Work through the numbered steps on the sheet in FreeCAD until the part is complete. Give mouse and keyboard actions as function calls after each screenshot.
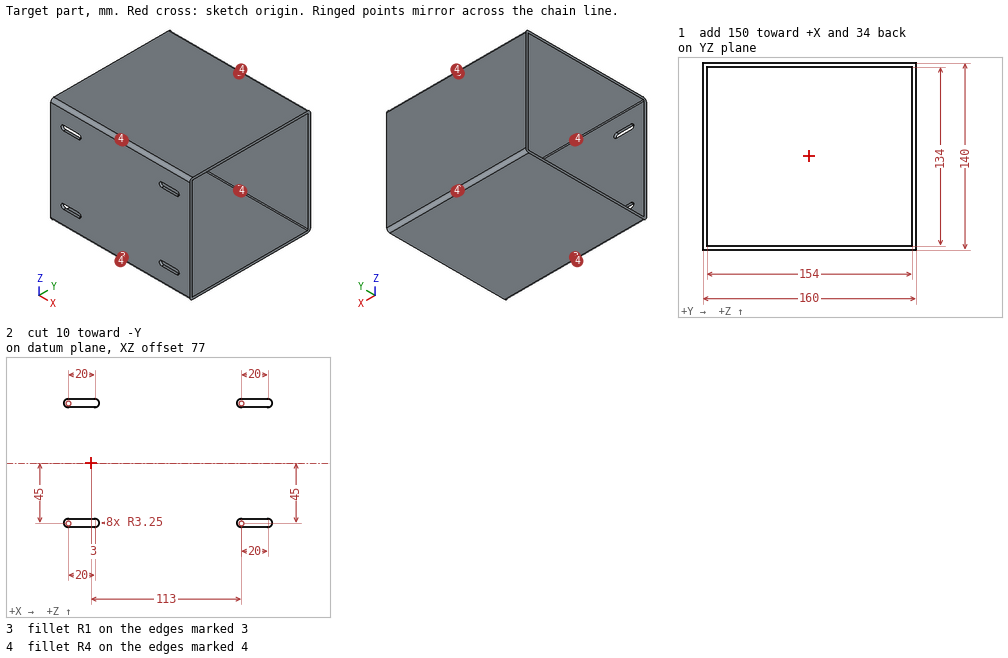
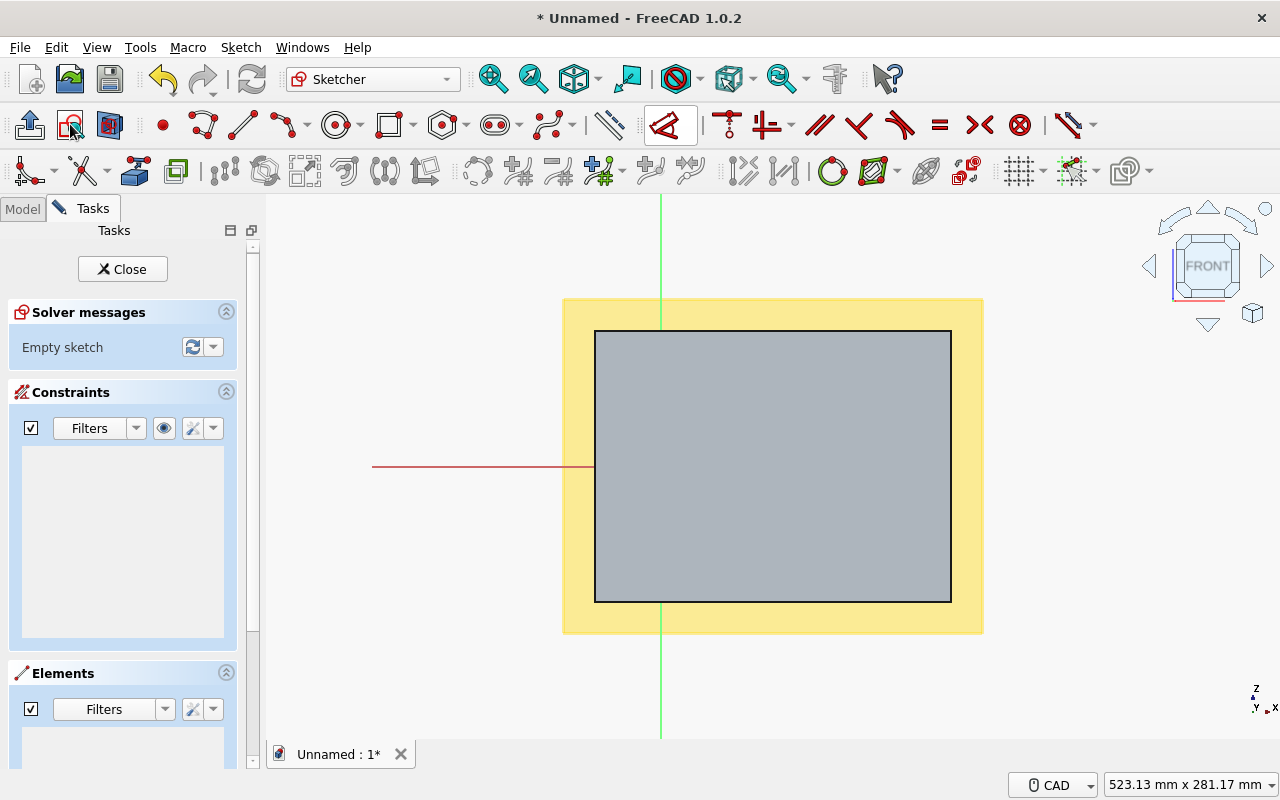
key(q)
key(s)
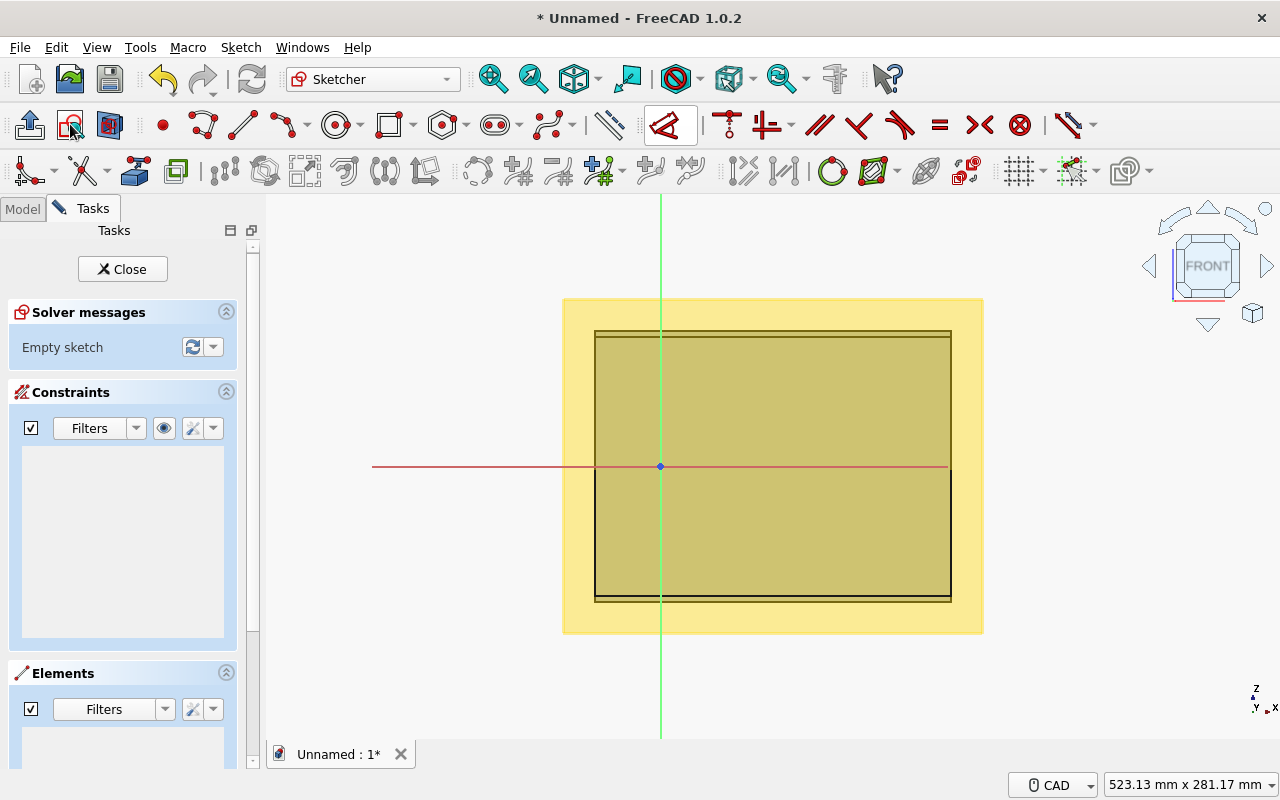
scroll(856, 466, up, 3)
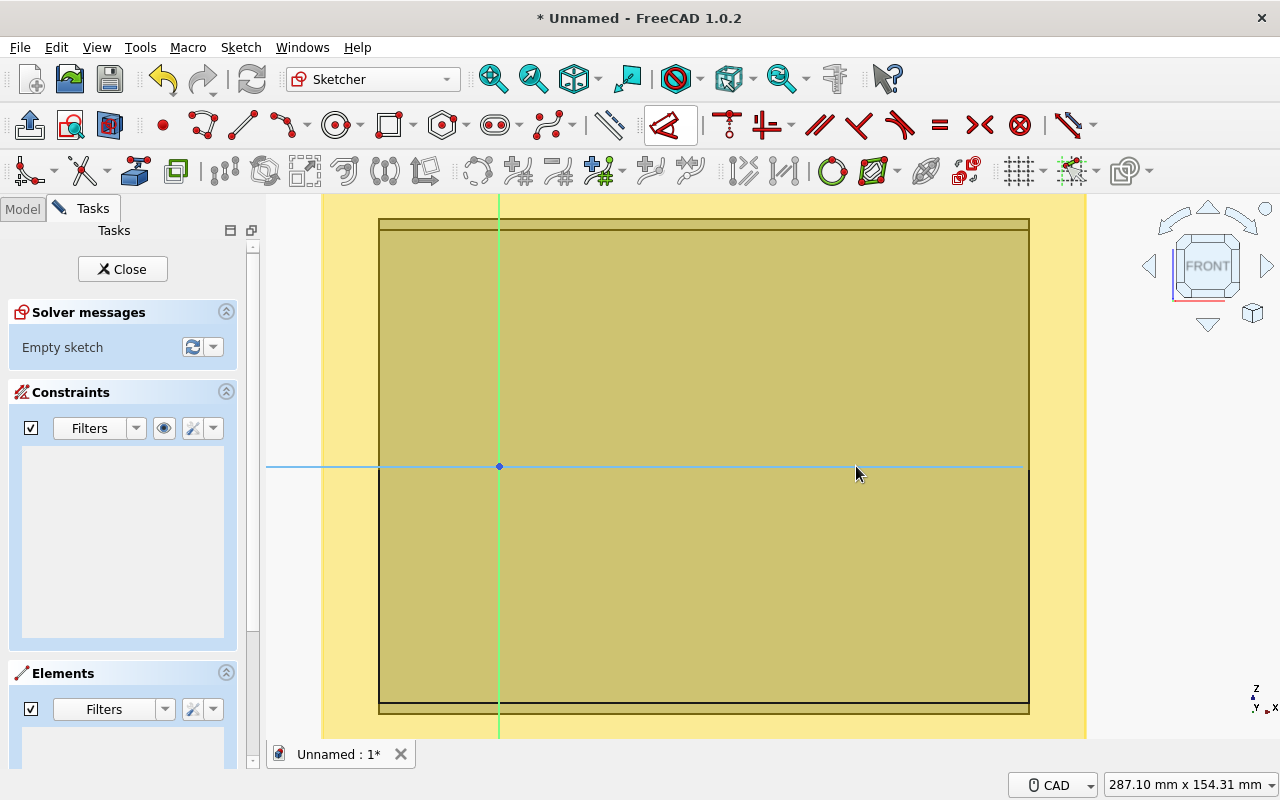
click(496, 126)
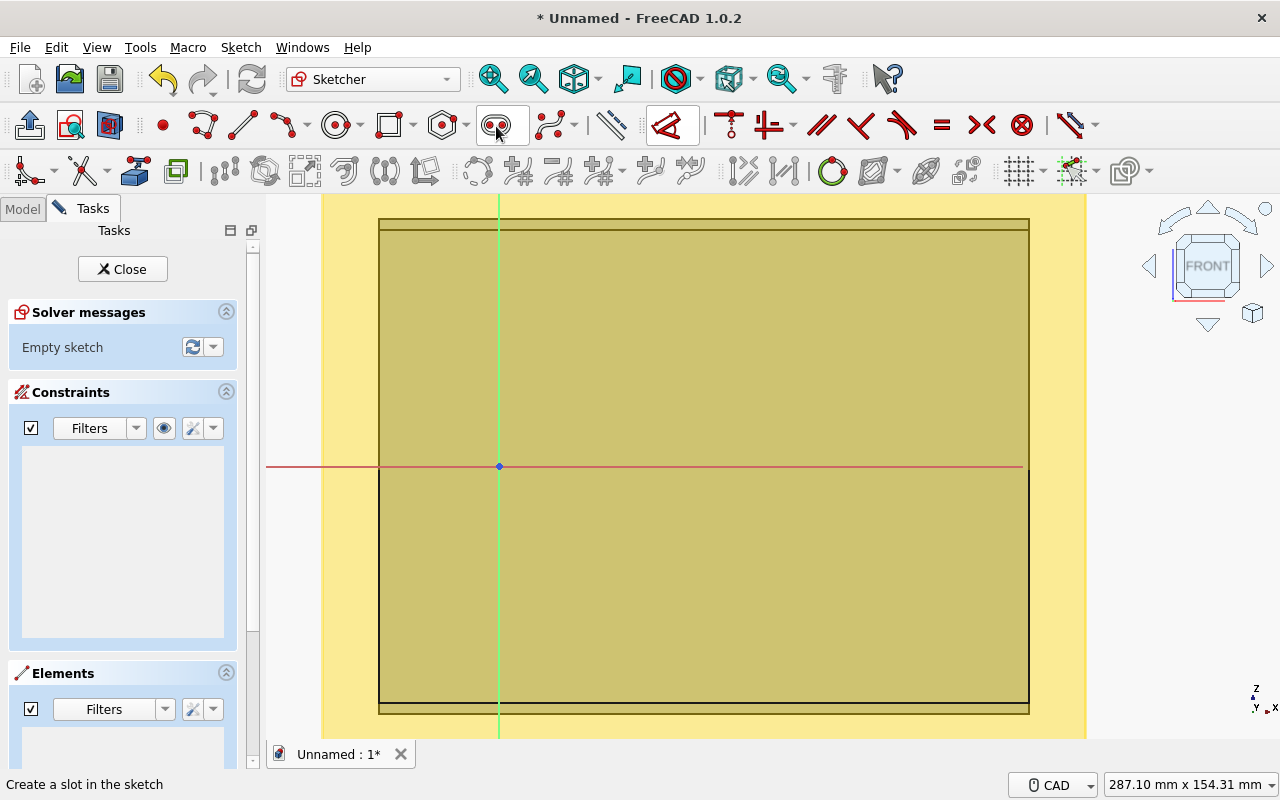
scroll(439, 625, up, 4)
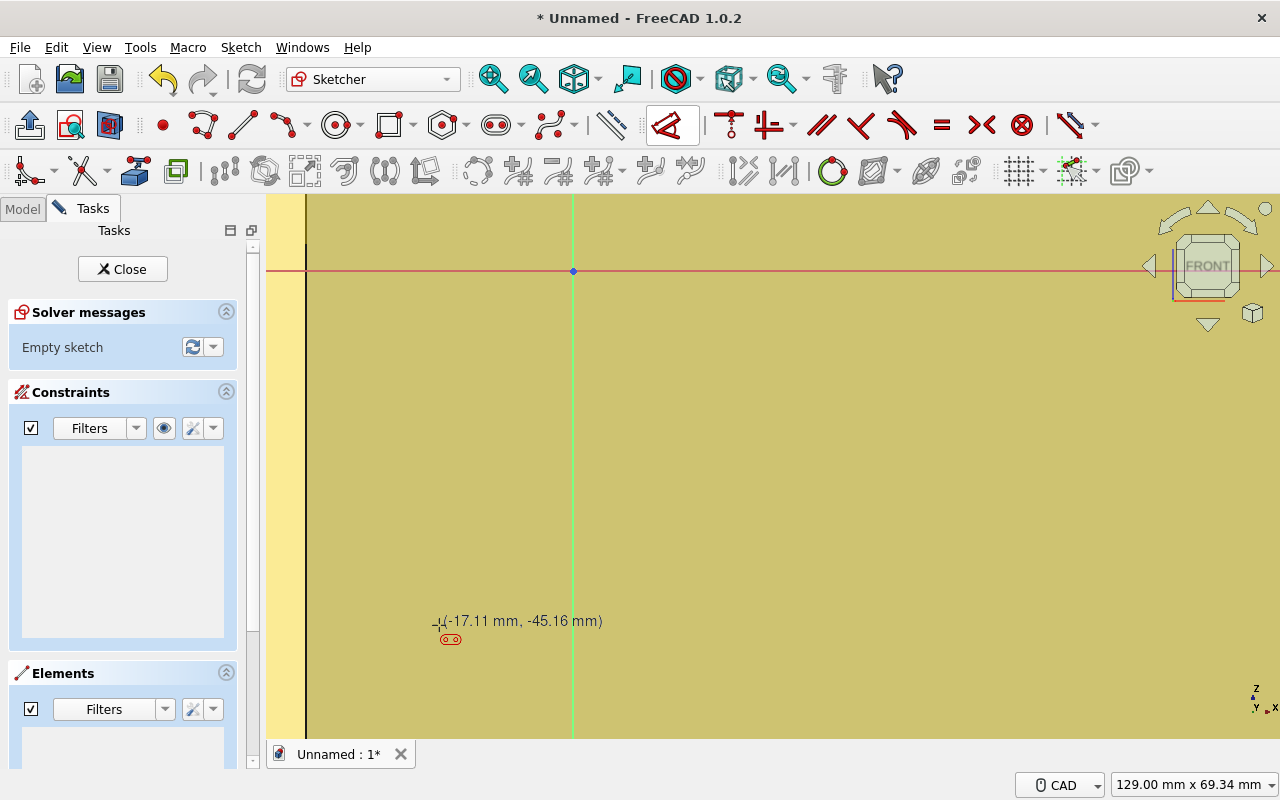
click(440, 625)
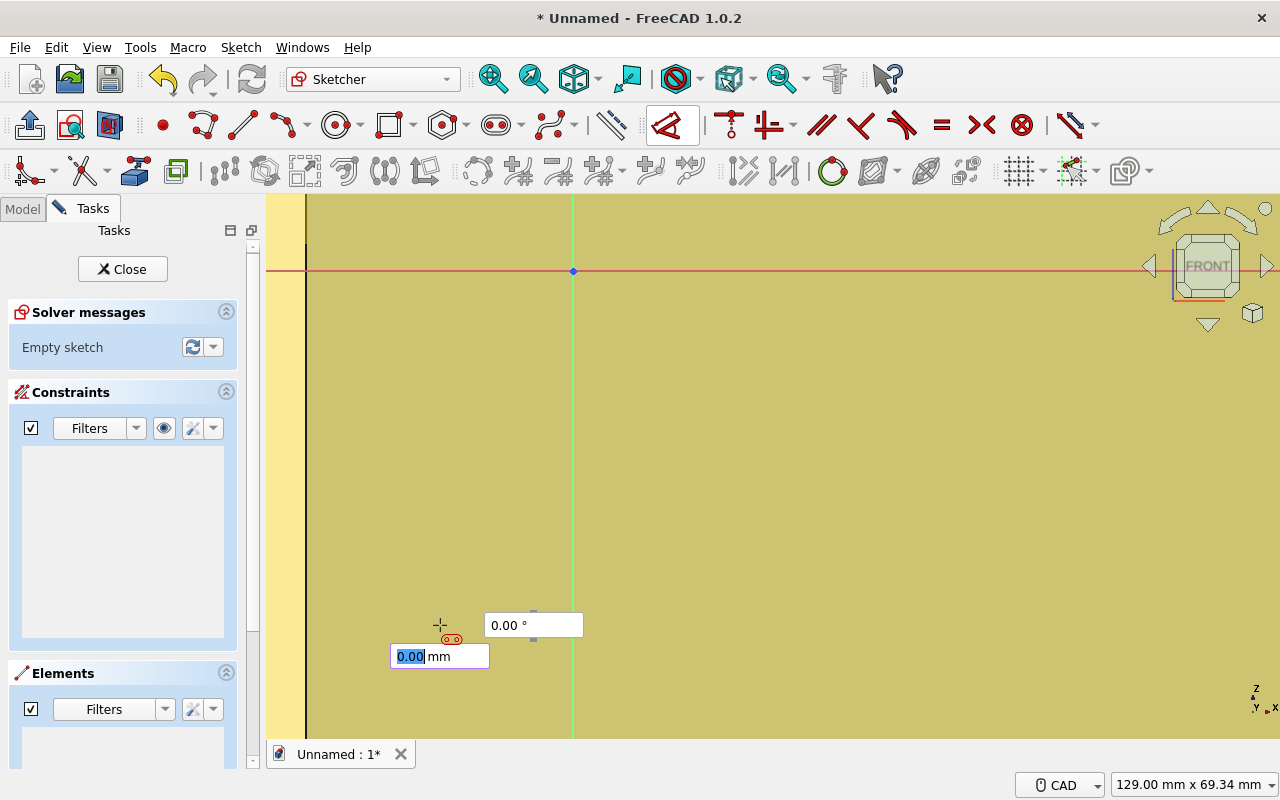
click(597, 625)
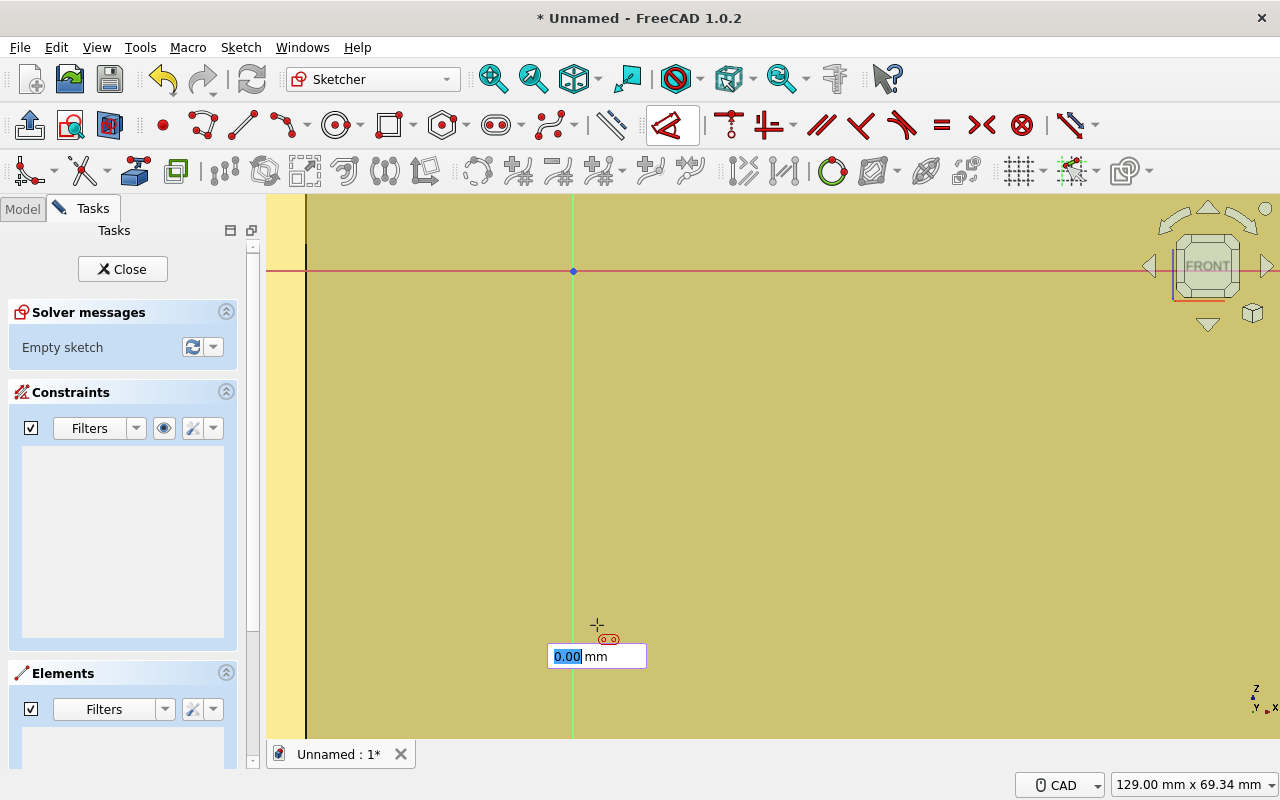
click(518, 651)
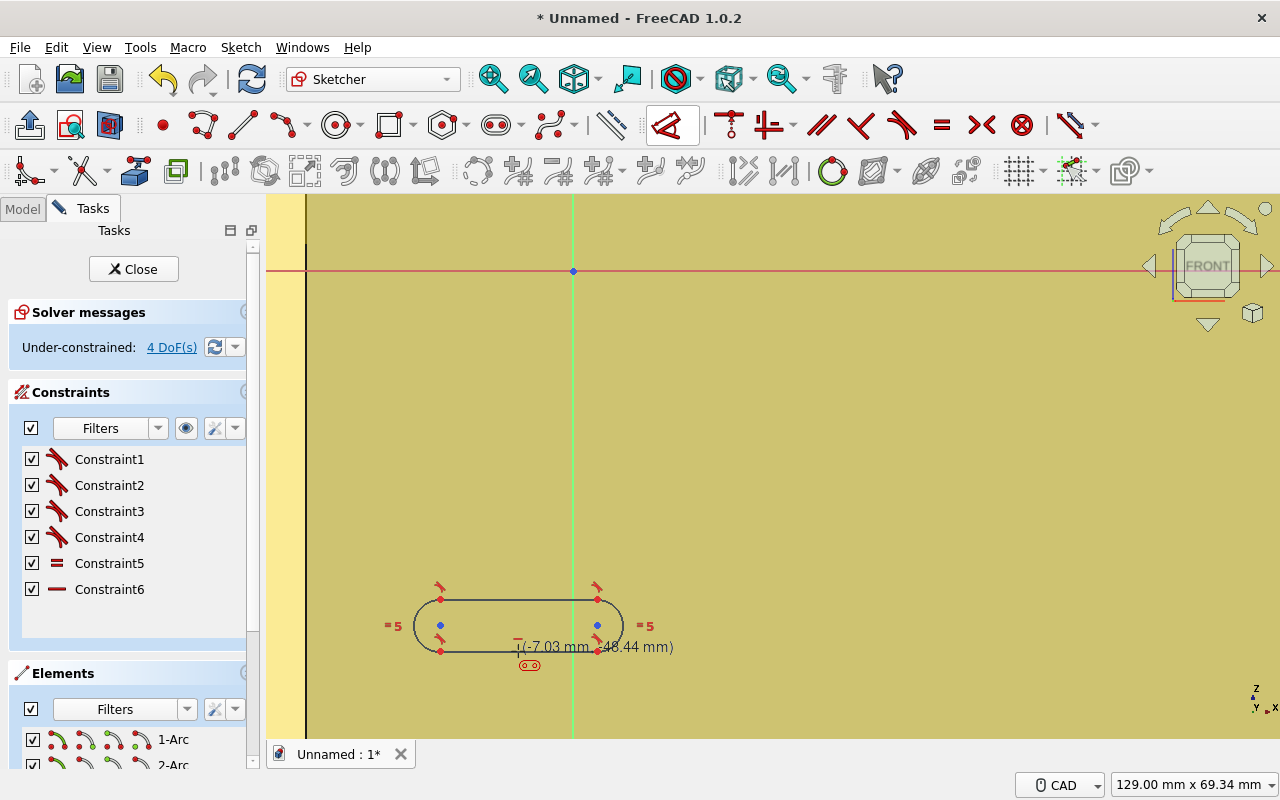
scroll(440, 626, down, 4)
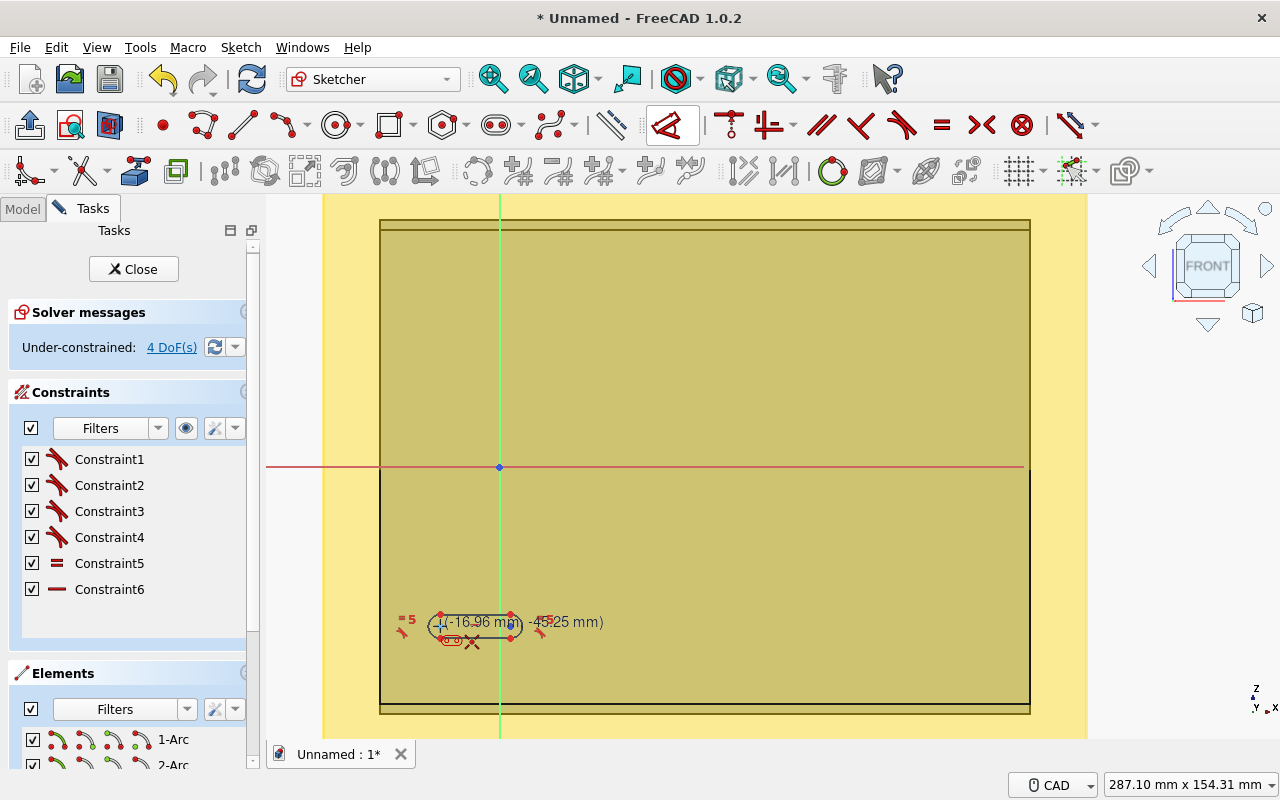
scroll(440, 308, up, 4)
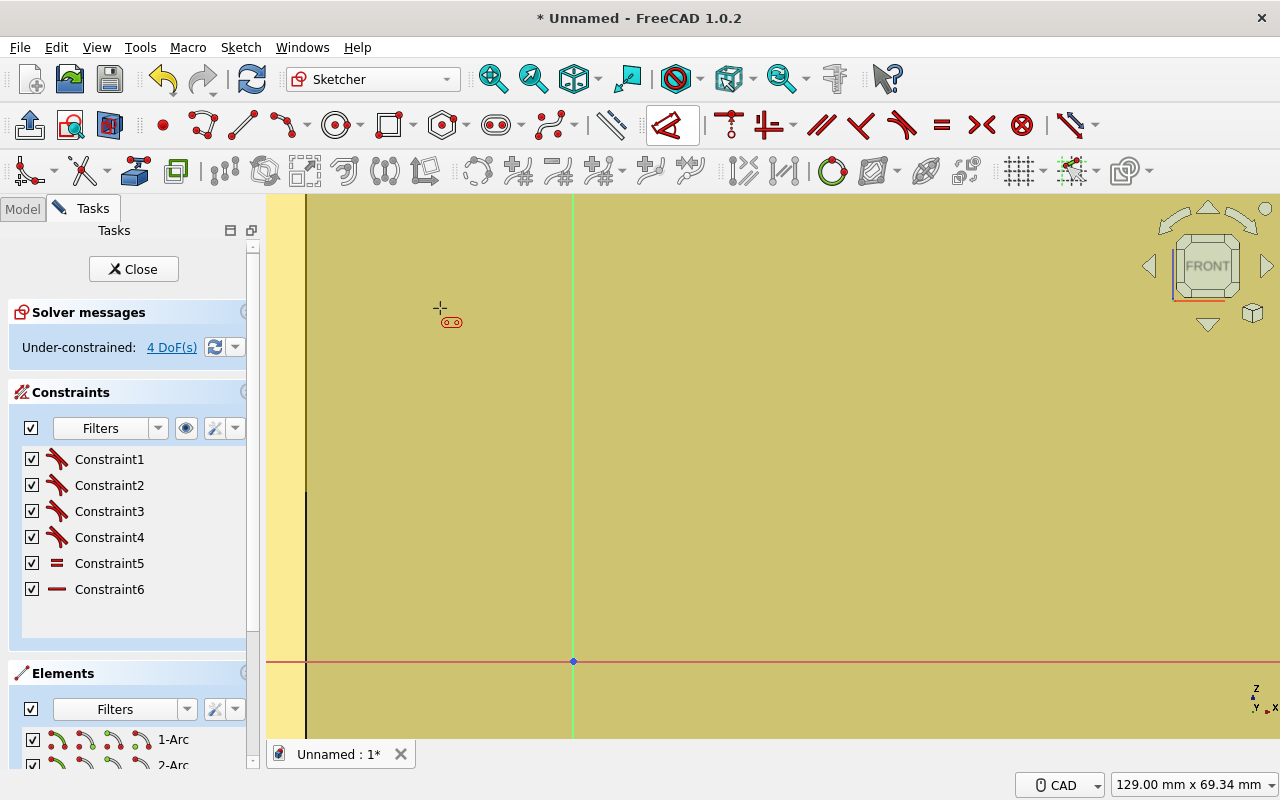
click(440, 308)